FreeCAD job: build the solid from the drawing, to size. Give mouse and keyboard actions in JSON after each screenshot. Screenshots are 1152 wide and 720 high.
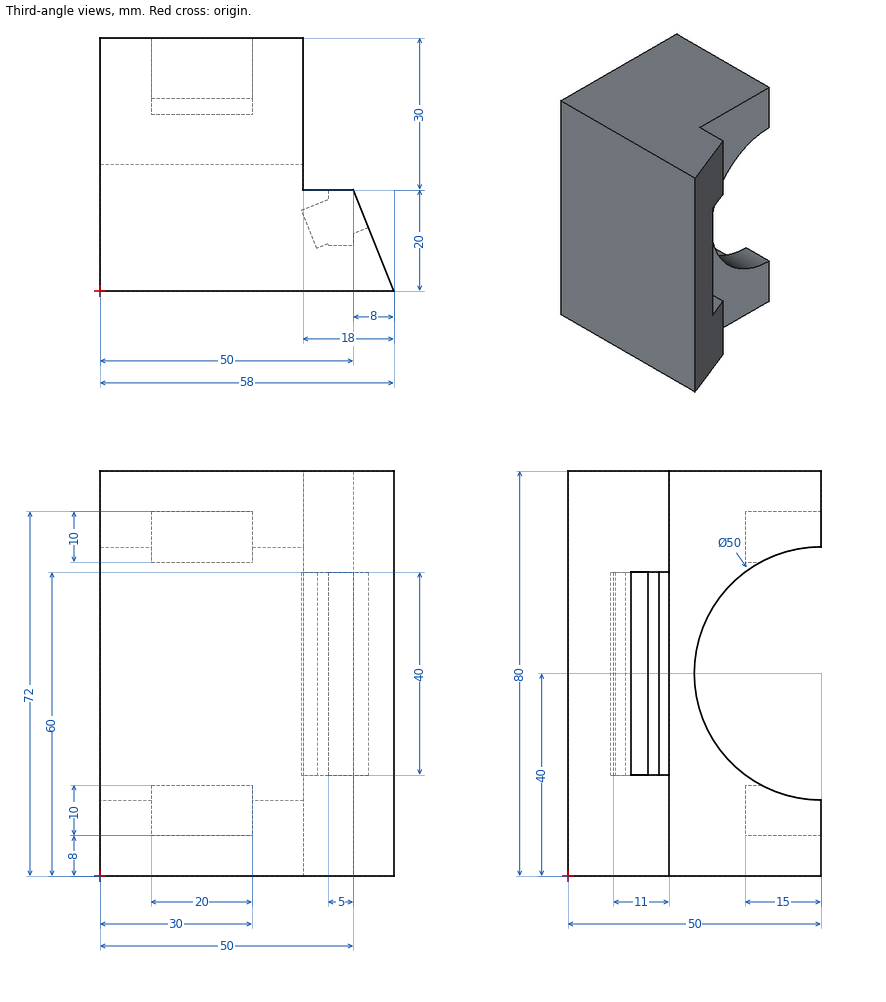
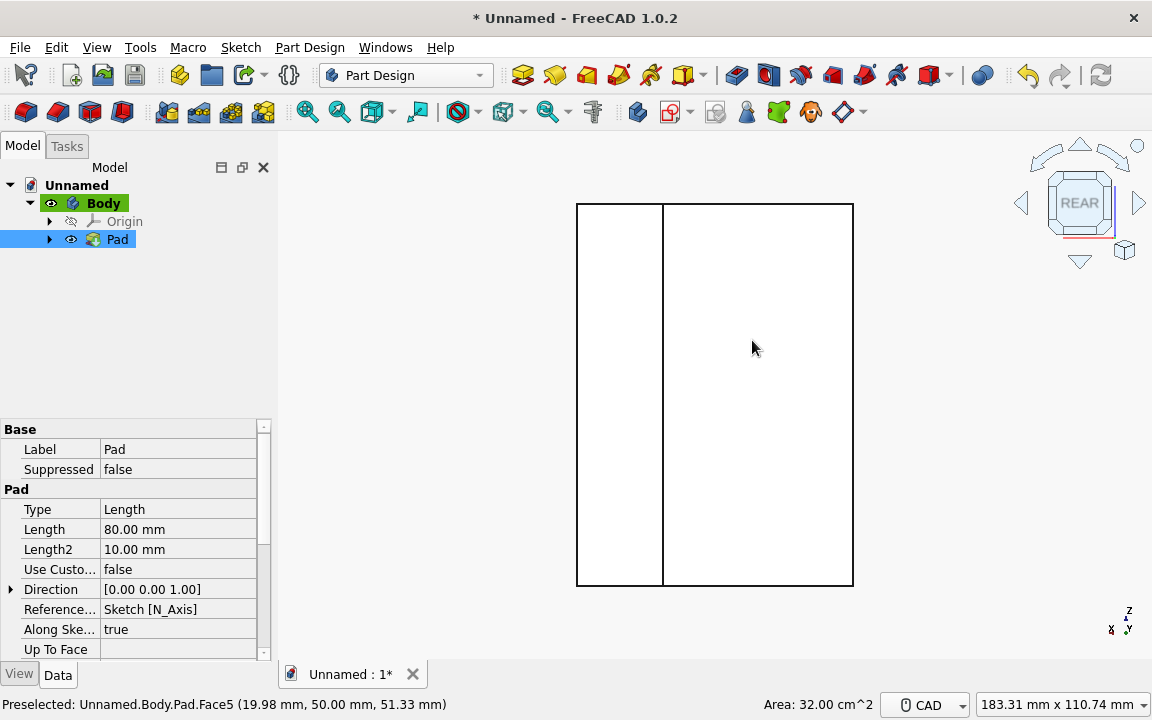
{"action": "left_click", "coordinate": [670, 112]}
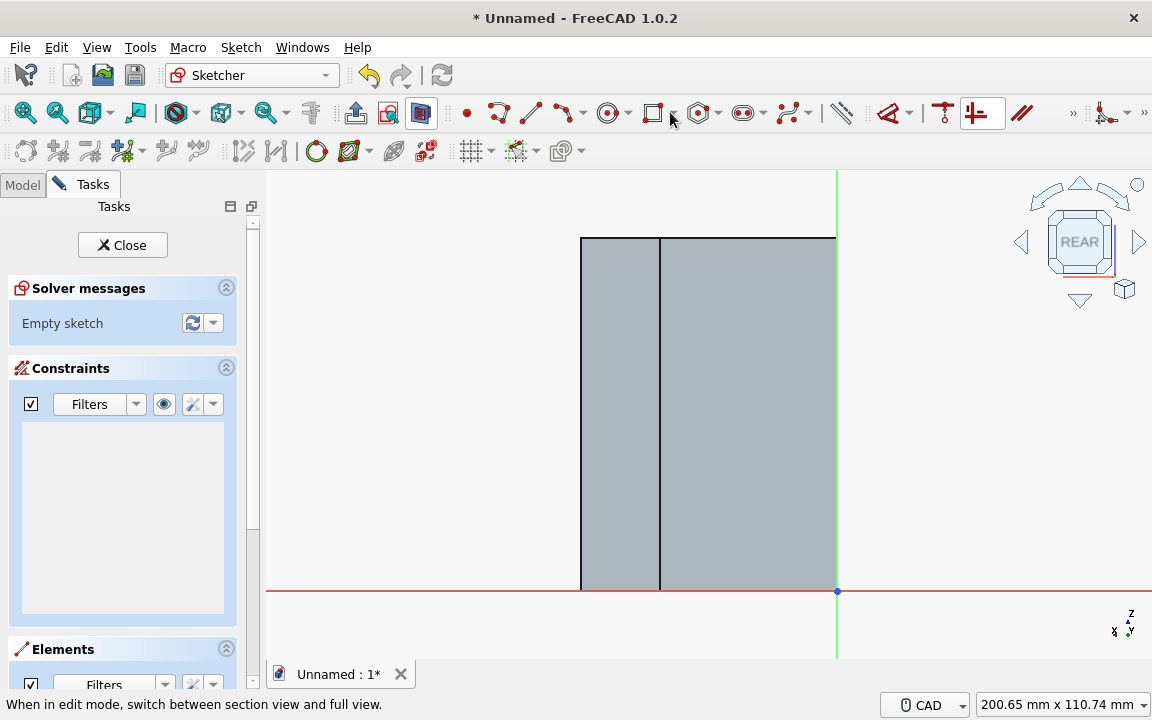
{"action": "left_click", "coordinate": [654, 114]}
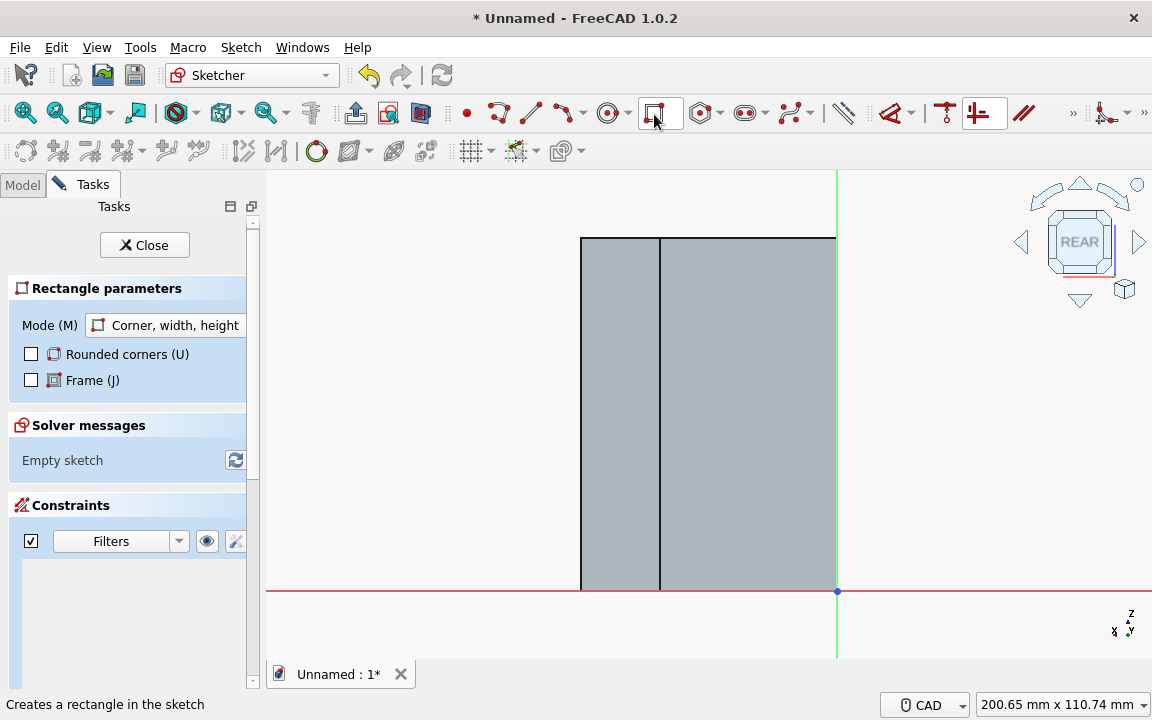
{"action": "left_click", "coordinate": [705, 512]}
{"action": "mouse_move", "coordinate": [793, 556]}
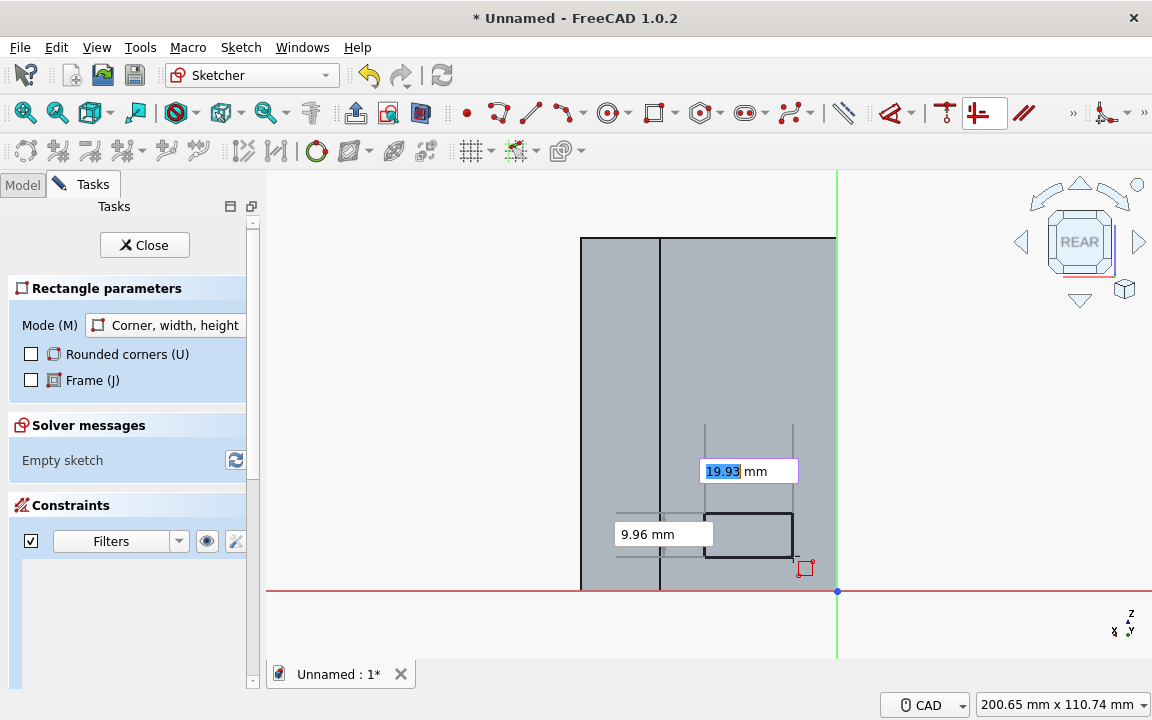
{"action": "type", "text": "20"}
{"action": "key", "text": "Tab"}
{"action": "type", "text": "10"}
{"action": "key", "text": "Return"}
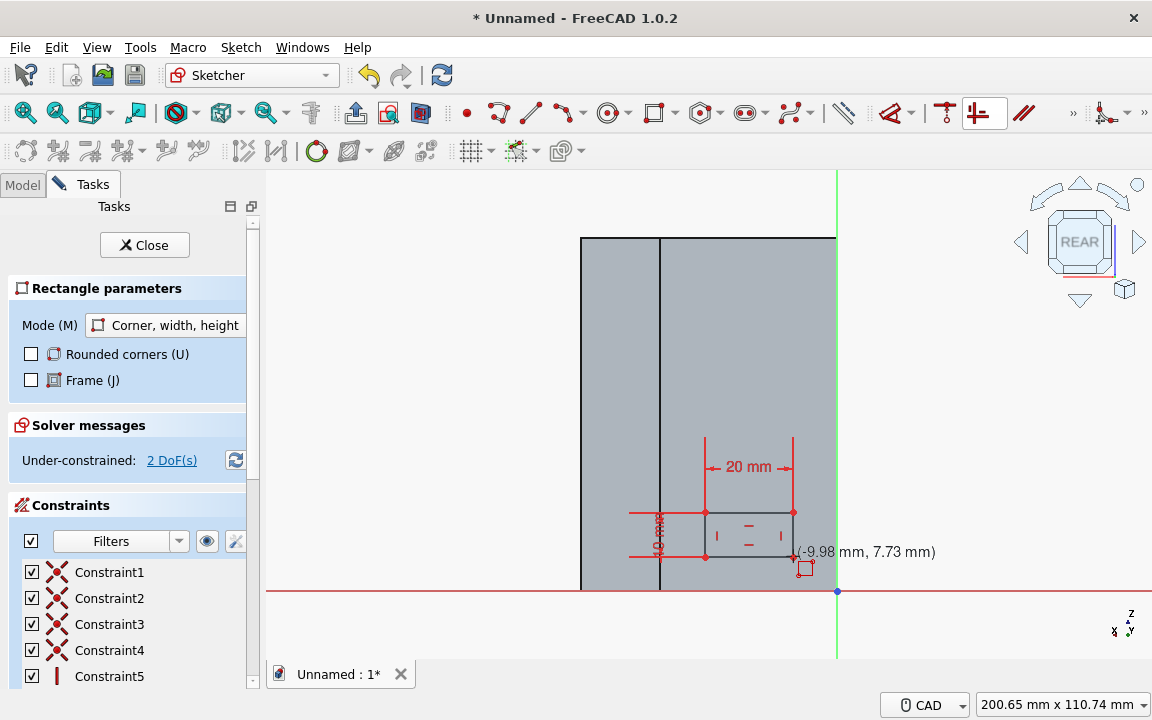
{"action": "left_click", "coordinate": [705, 273]}
{"action": "mouse_move", "coordinate": [793, 317]}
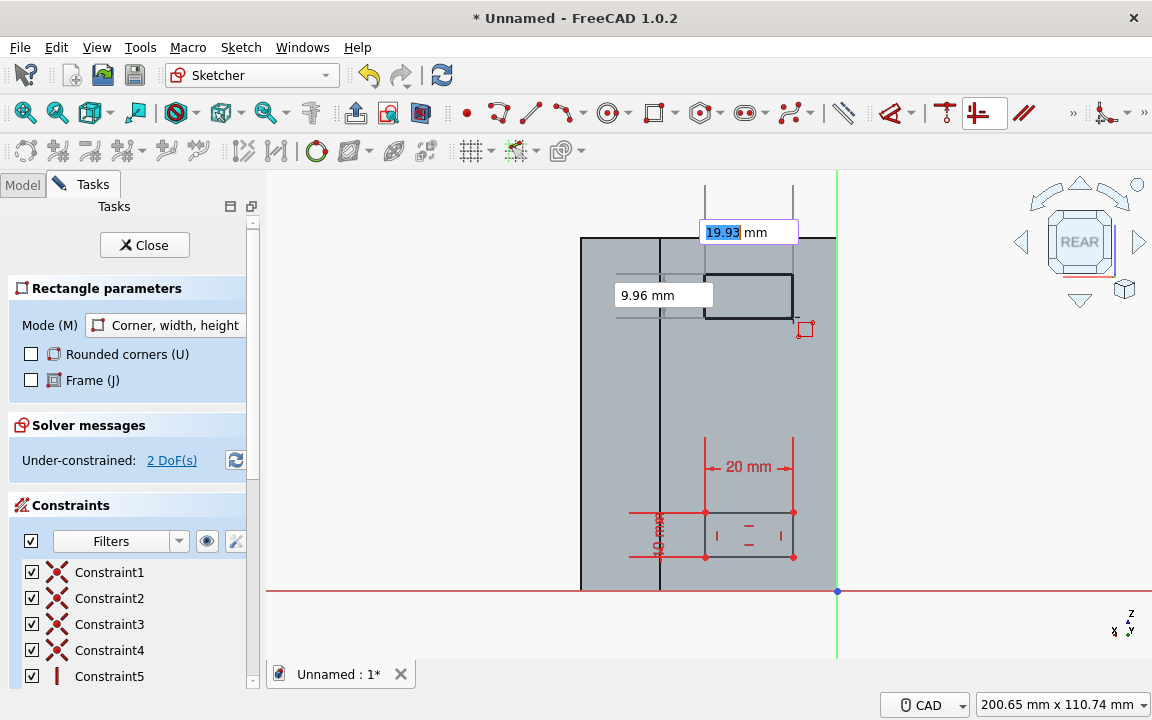
{"action": "type", "text": "20"}
{"action": "key", "text": "Tab"}
{"action": "type", "text": "10"}
{"action": "key", "text": "Return"}
{"action": "key", "text": "Escape"}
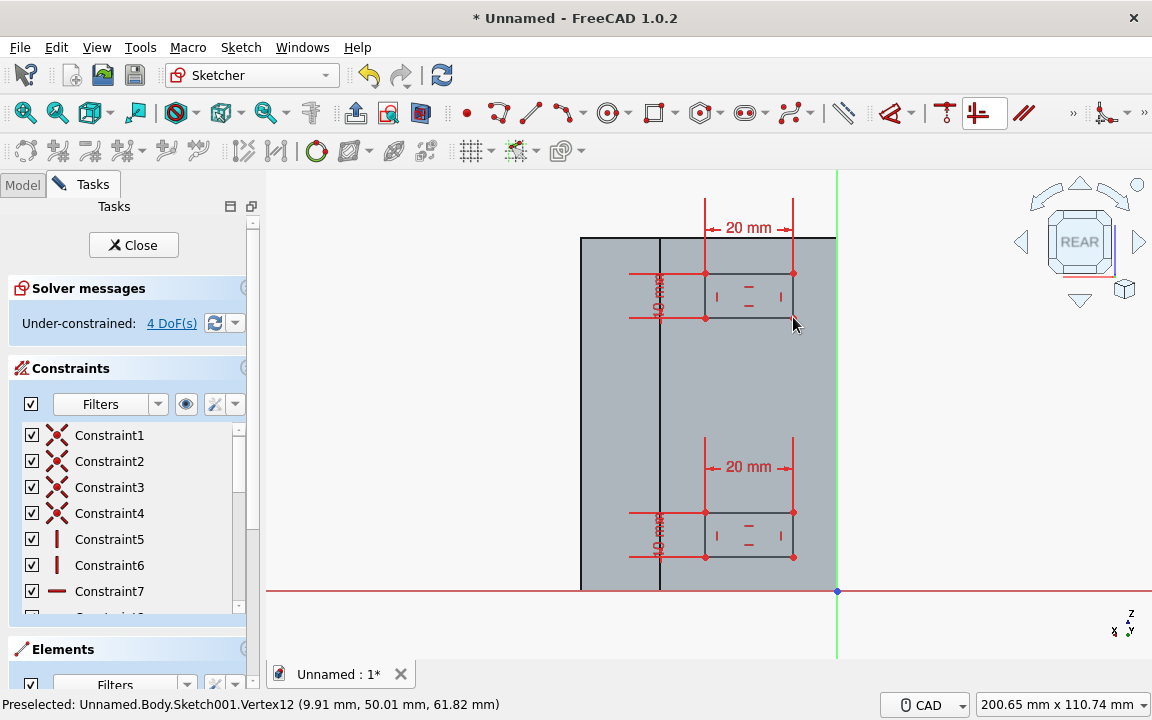
{"action": "left_click", "coordinate": [890, 114]}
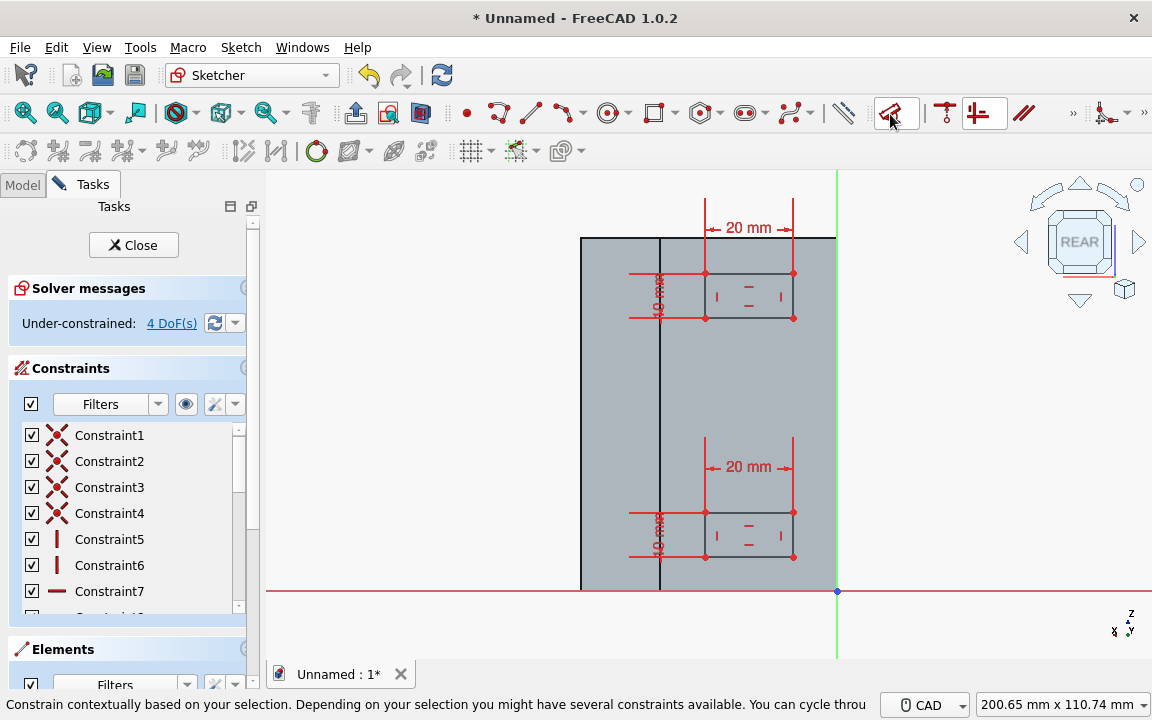
{"action": "left_click", "coordinate": [705, 557]}
{"action": "left_click", "coordinate": [871, 574]}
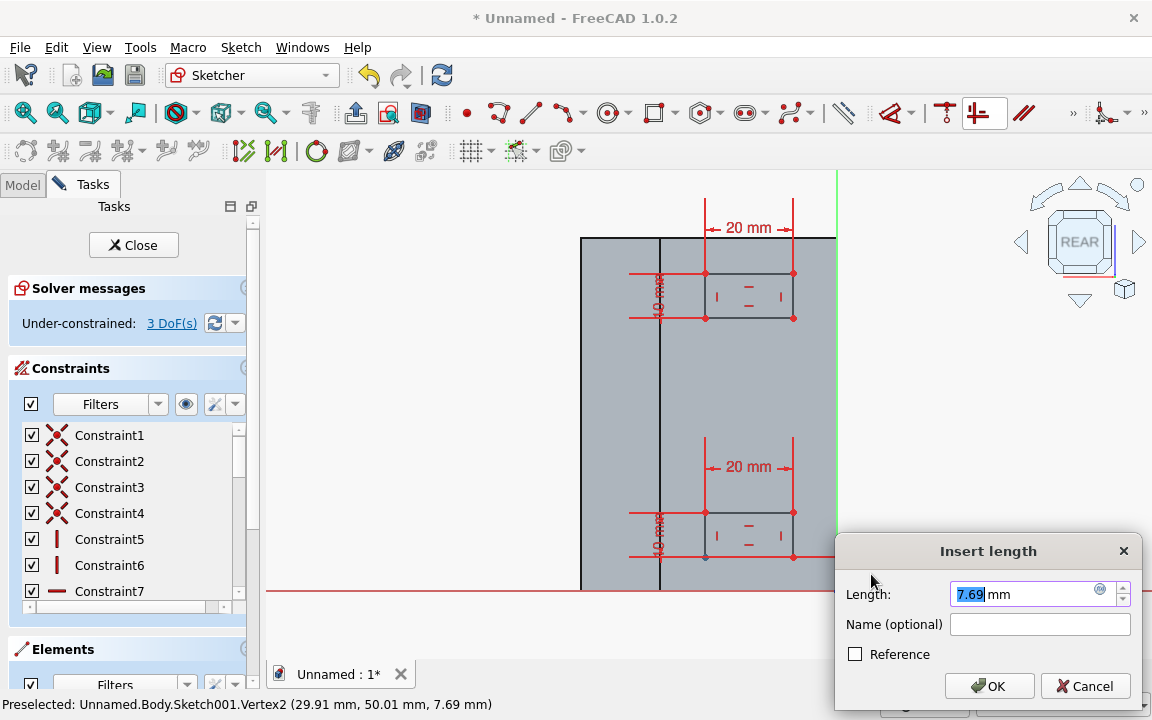
{"action": "type", "text": "8"}
{"action": "key", "text": "Return"}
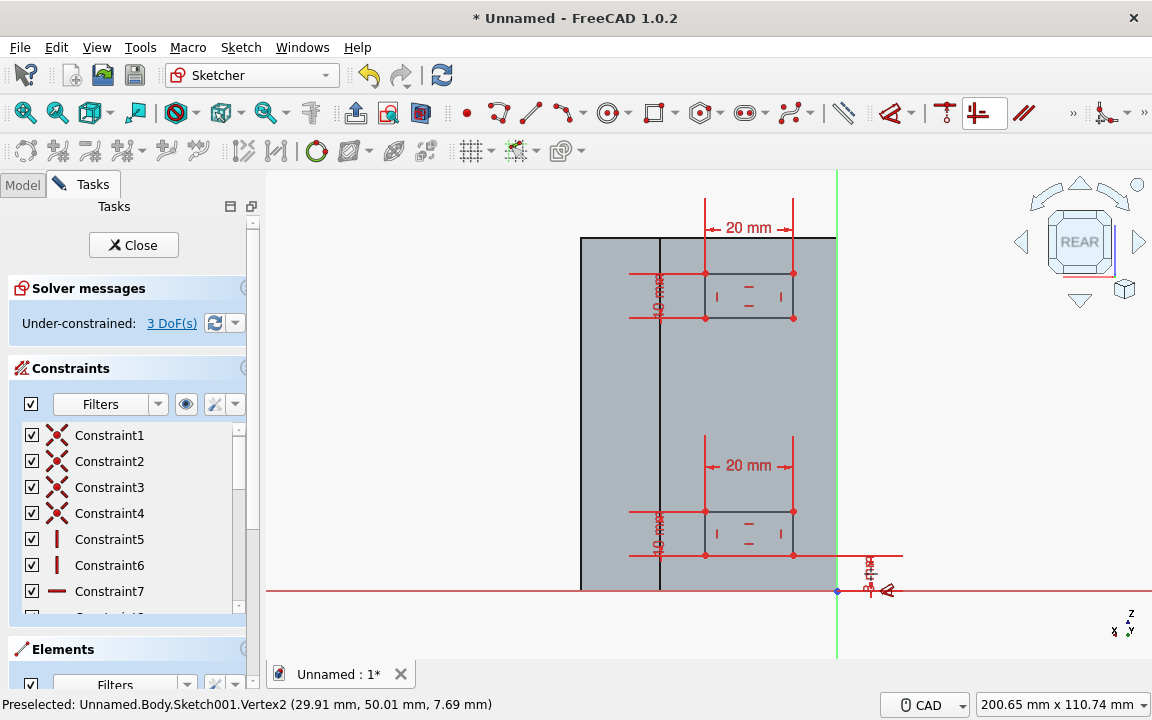
{"action": "left_click", "coordinate": [705, 512]}
{"action": "left_click", "coordinate": [771, 625]}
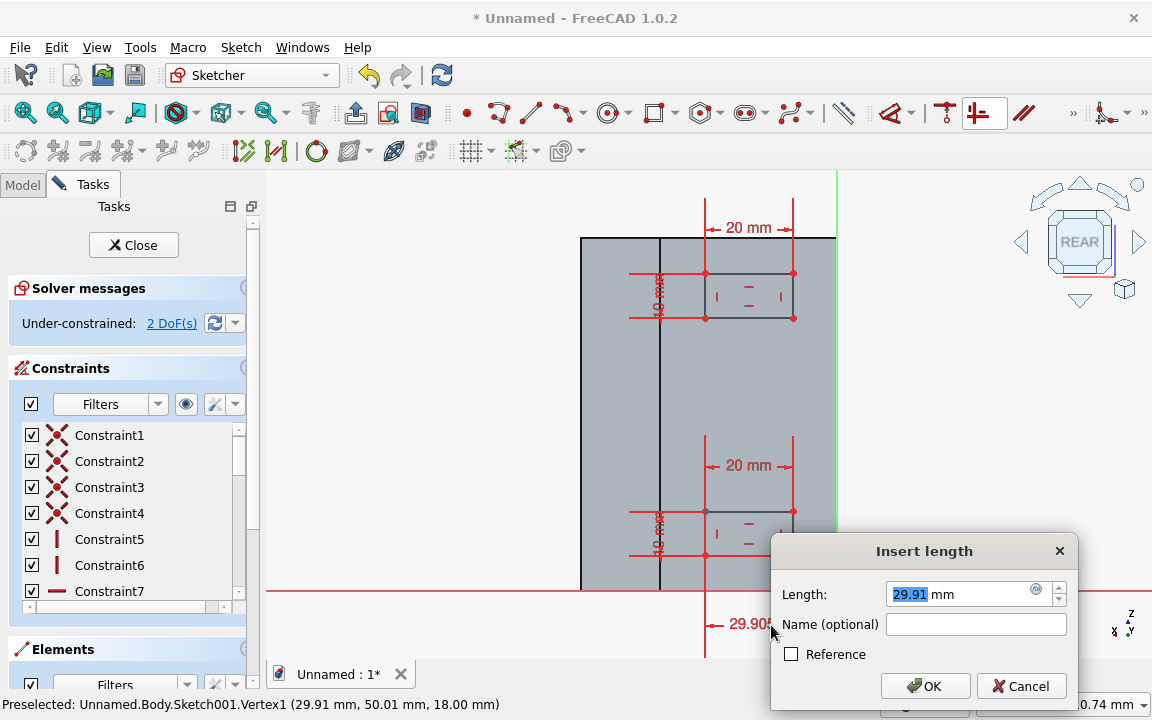
{"action": "type", "text": "30"}
{"action": "key", "text": "Return"}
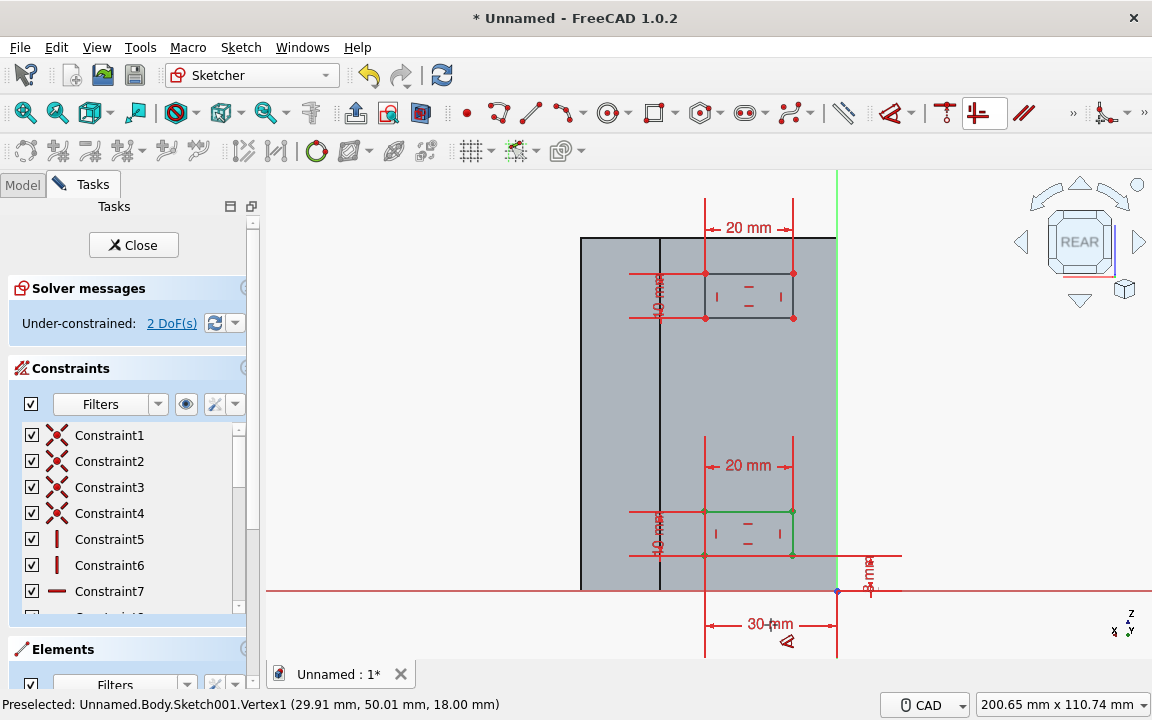
{"action": "left_click", "coordinate": [705, 274]}
{"action": "left_click", "coordinate": [771, 240]}